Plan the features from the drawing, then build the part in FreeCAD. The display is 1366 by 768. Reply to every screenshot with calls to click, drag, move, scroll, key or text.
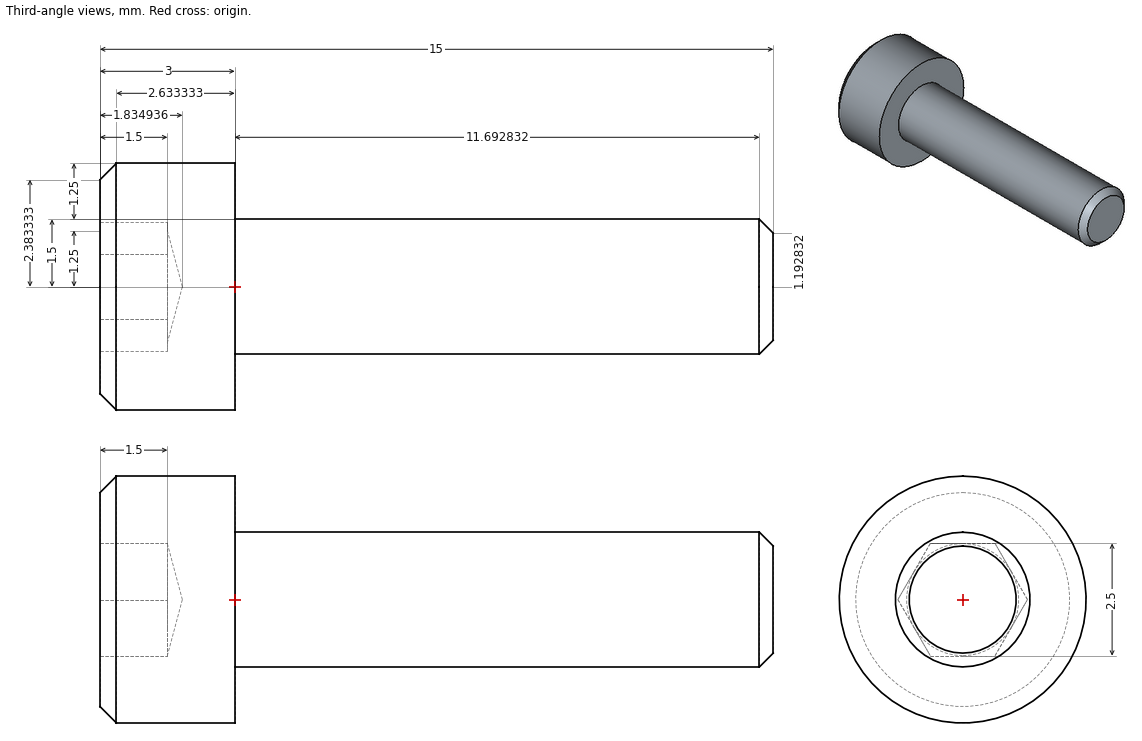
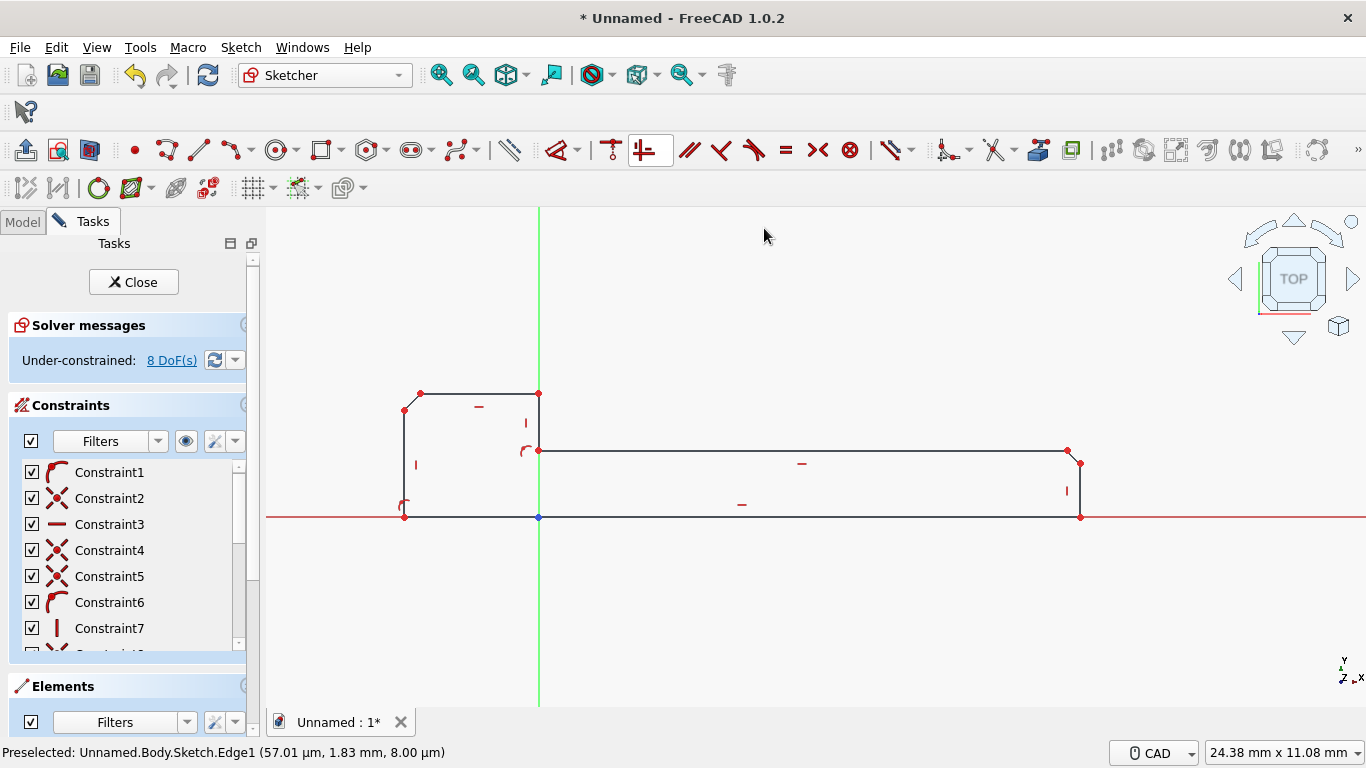
click(607, 517)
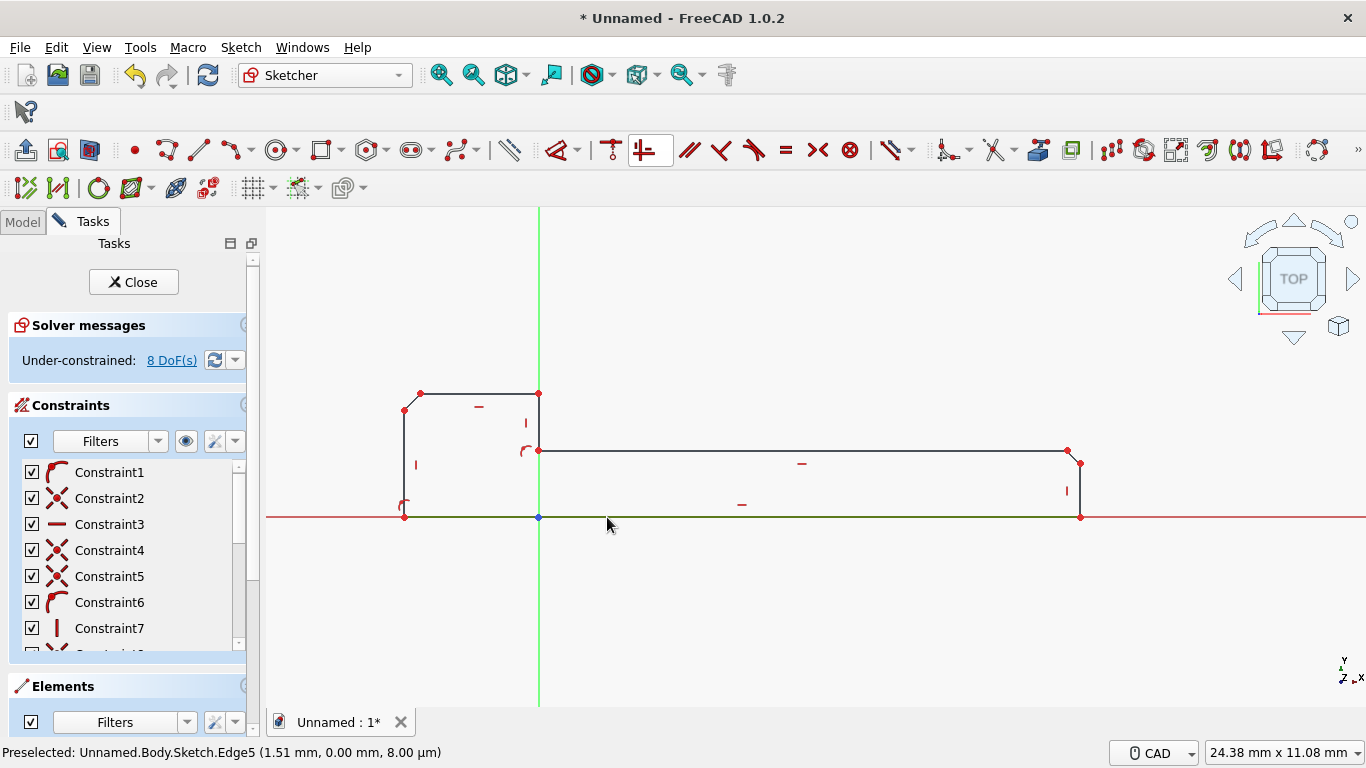
key(l)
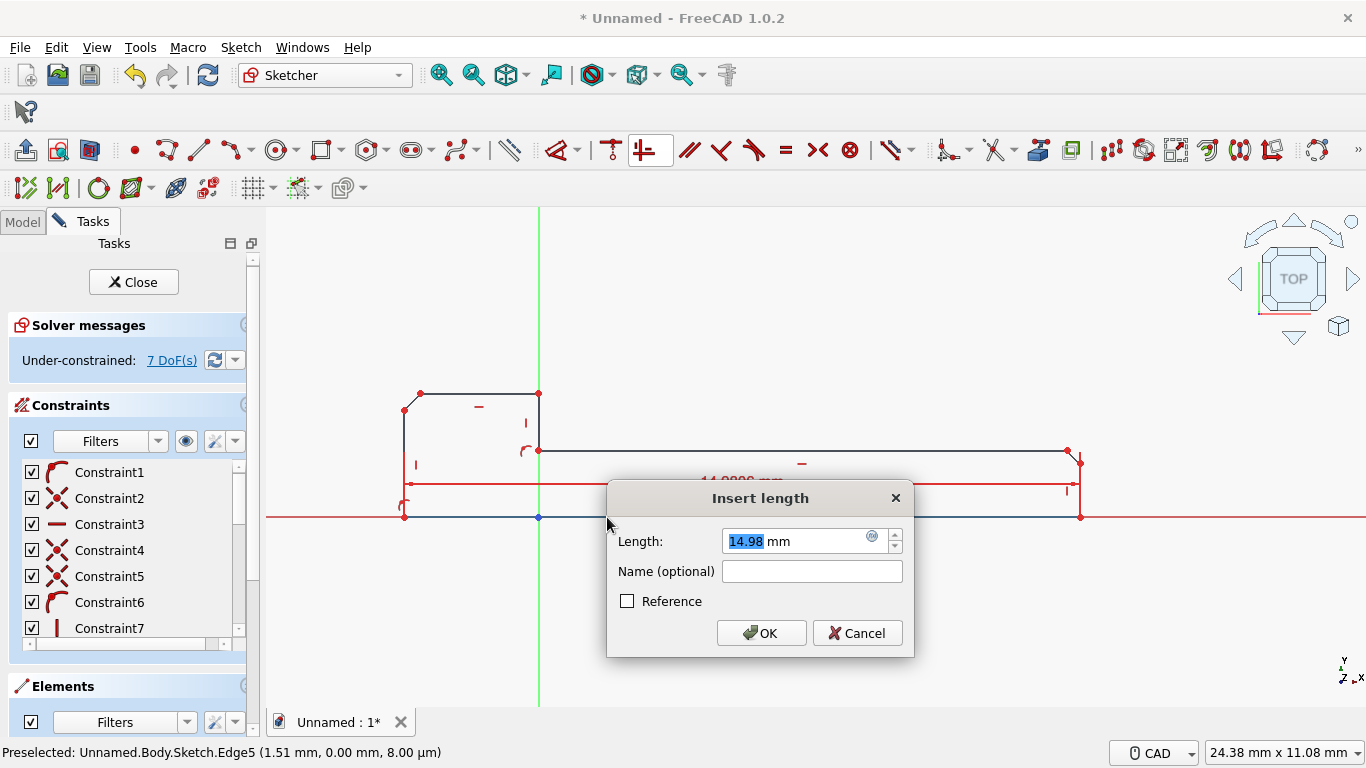
text(15)
key(Return)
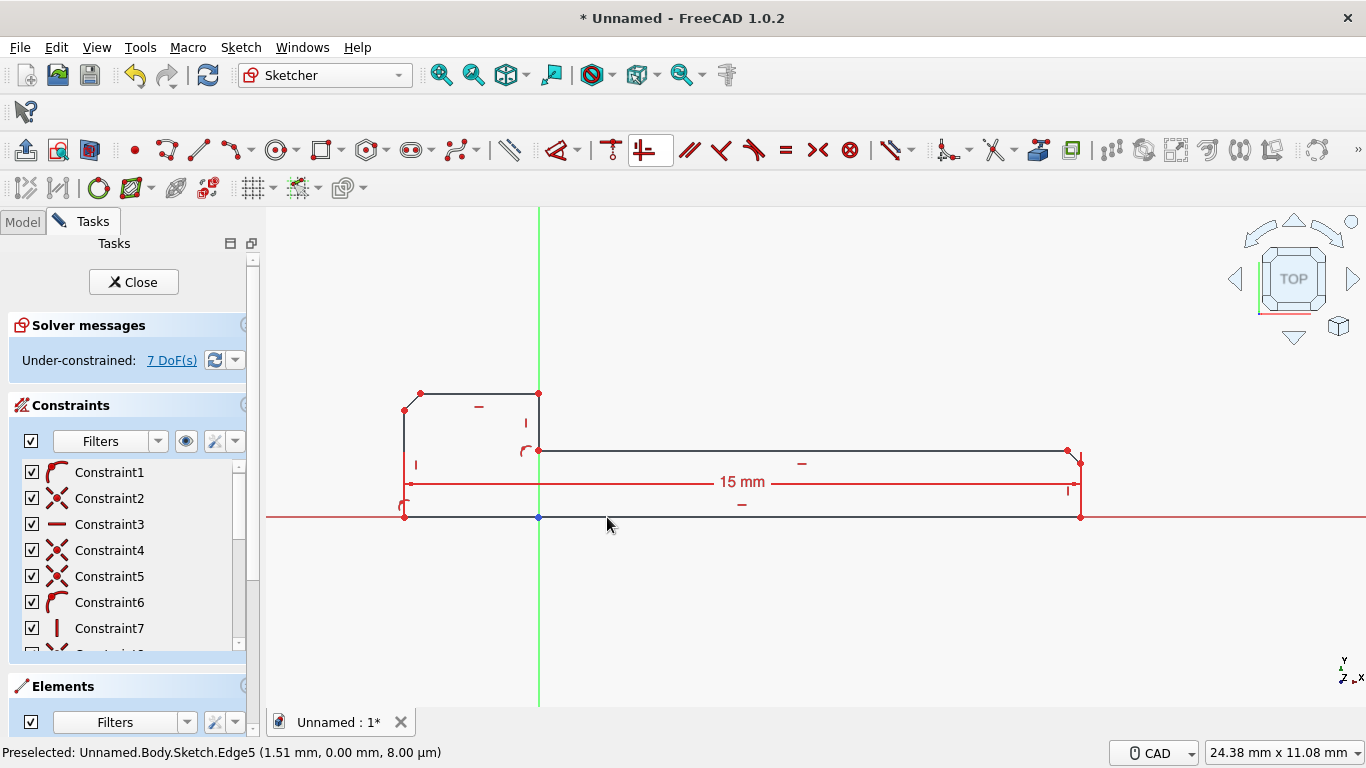
click(404, 411)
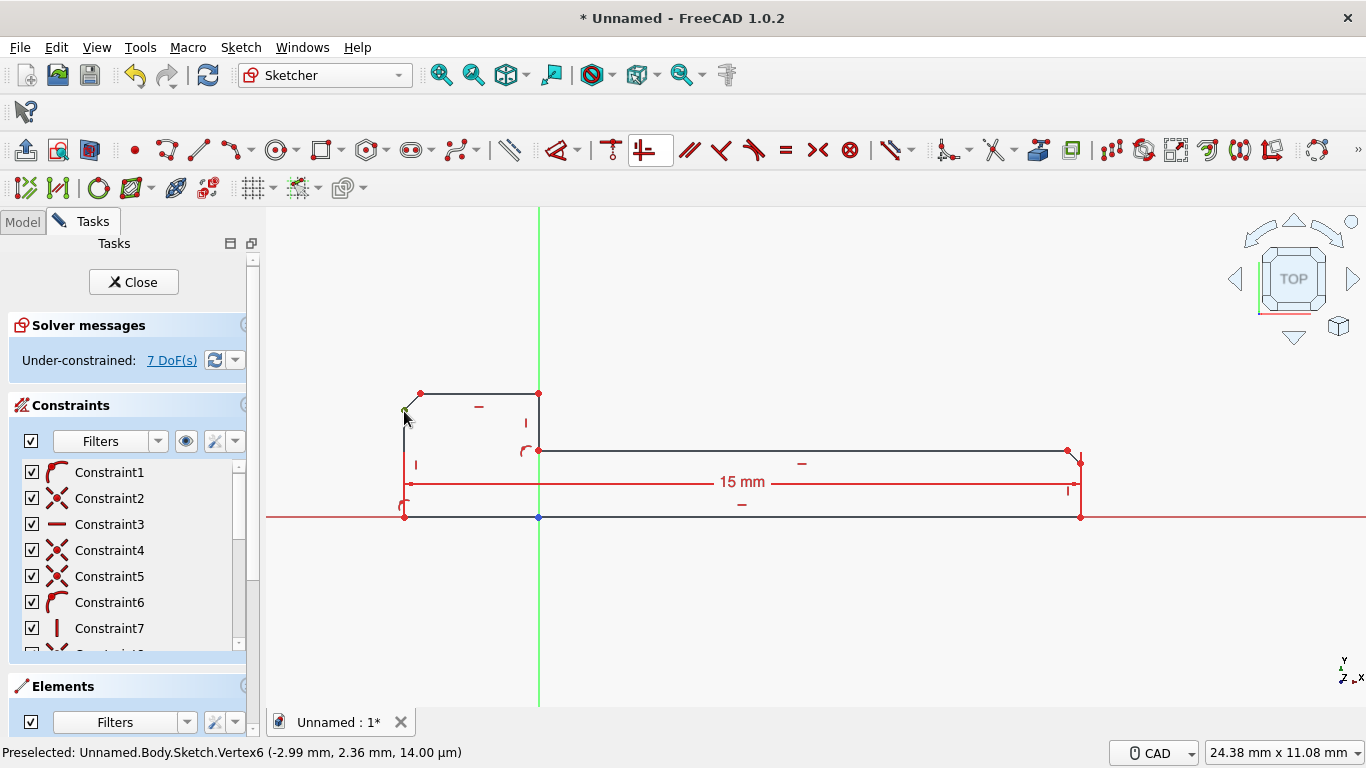
click(580, 150)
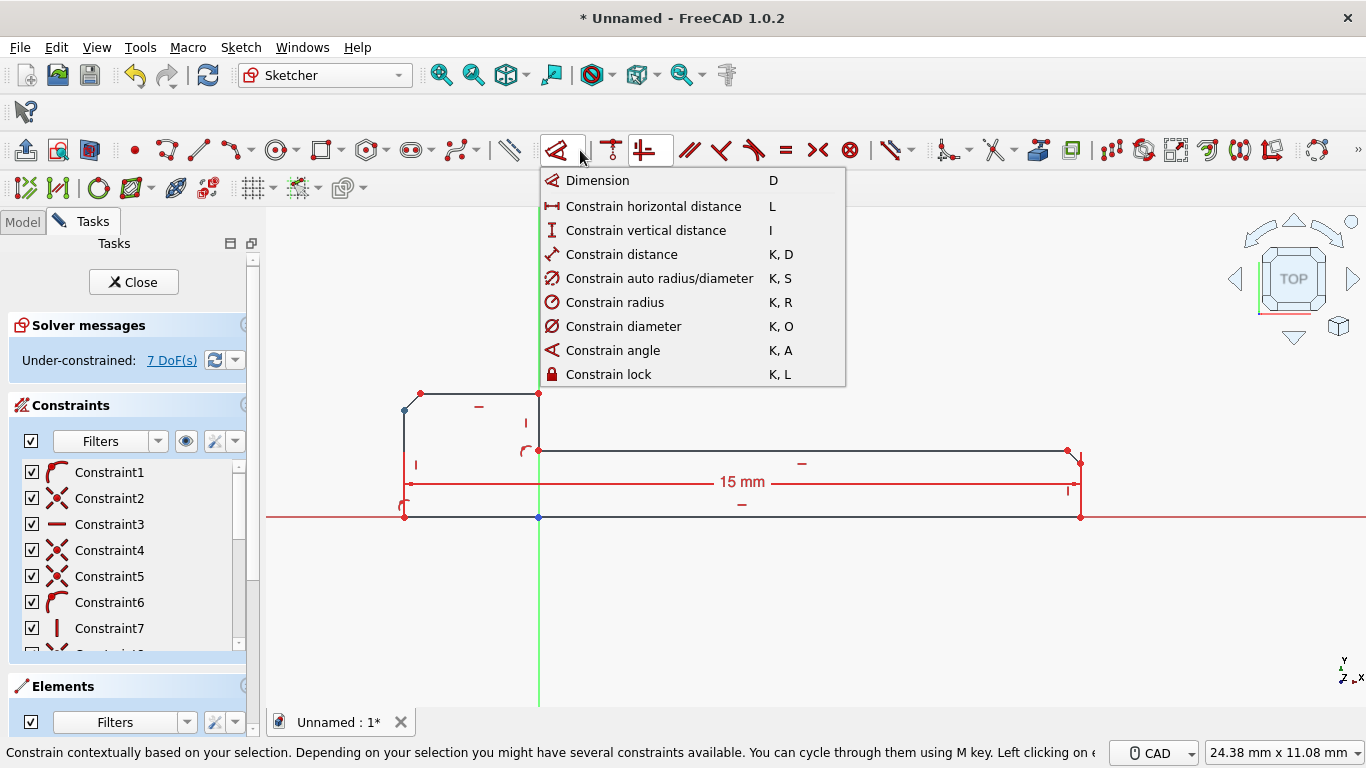
click(693, 206)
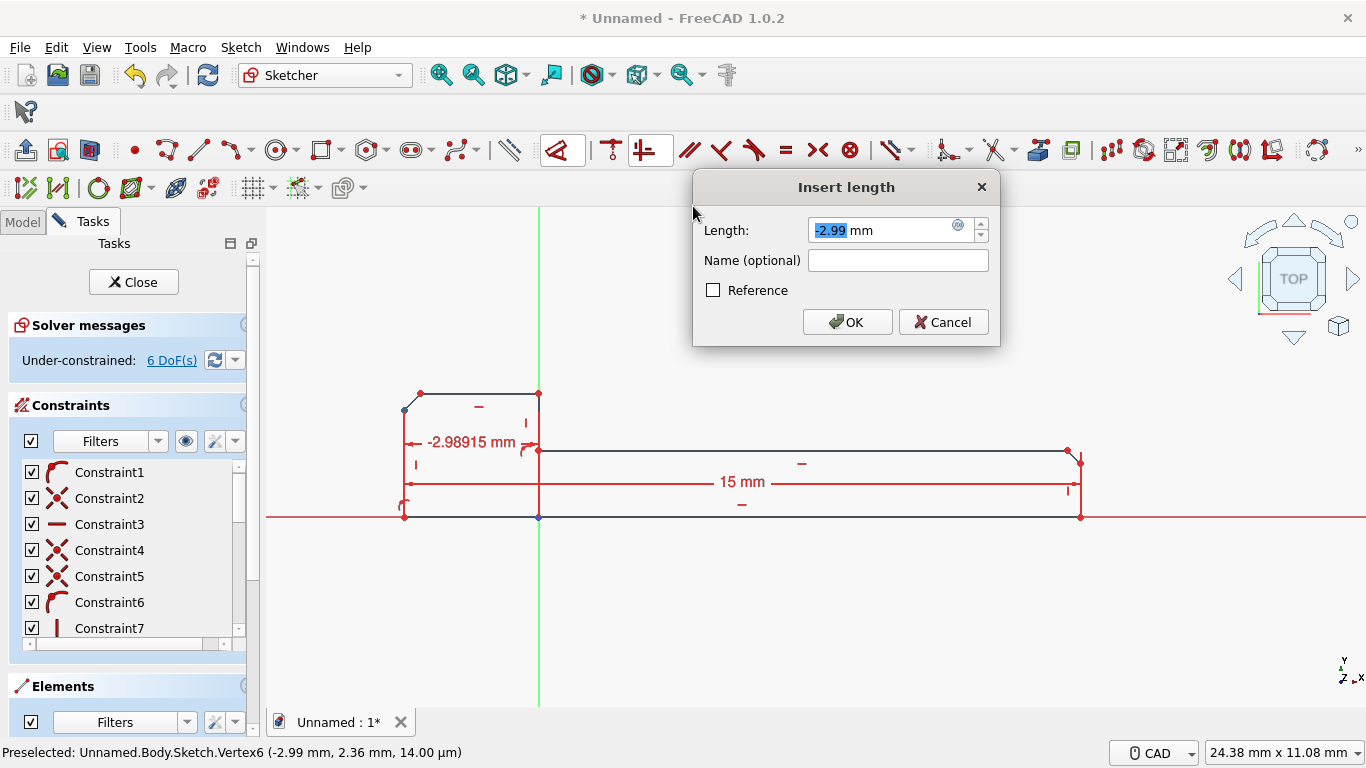
text(-3)
key(Return)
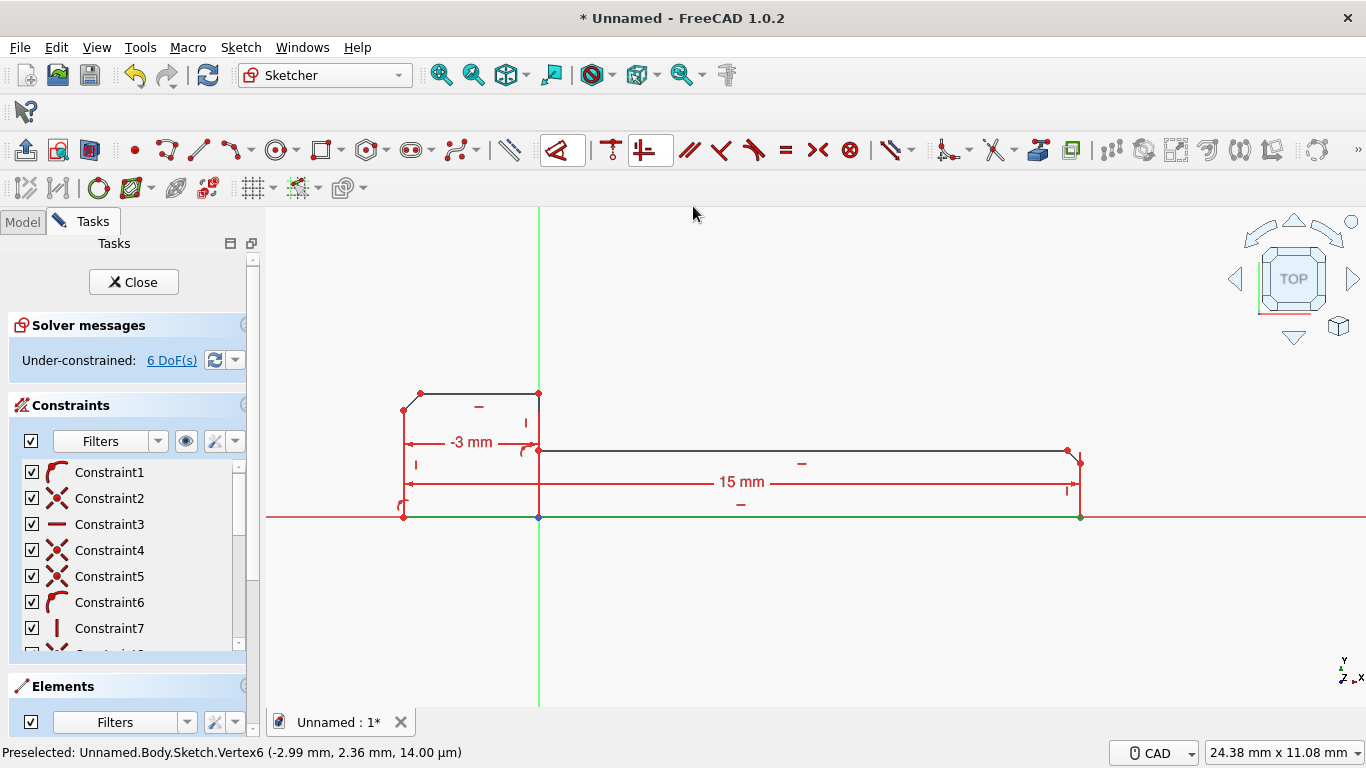
click(539, 434)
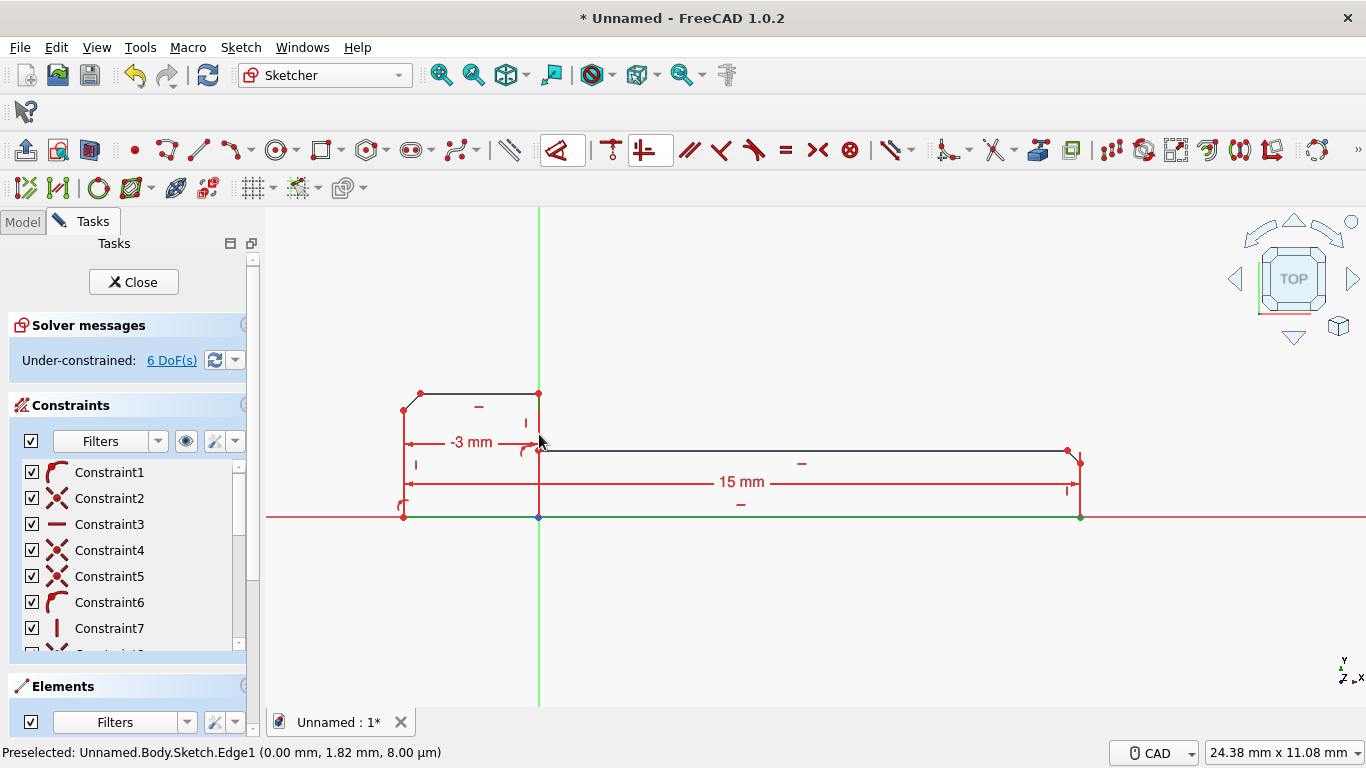
click(580, 150)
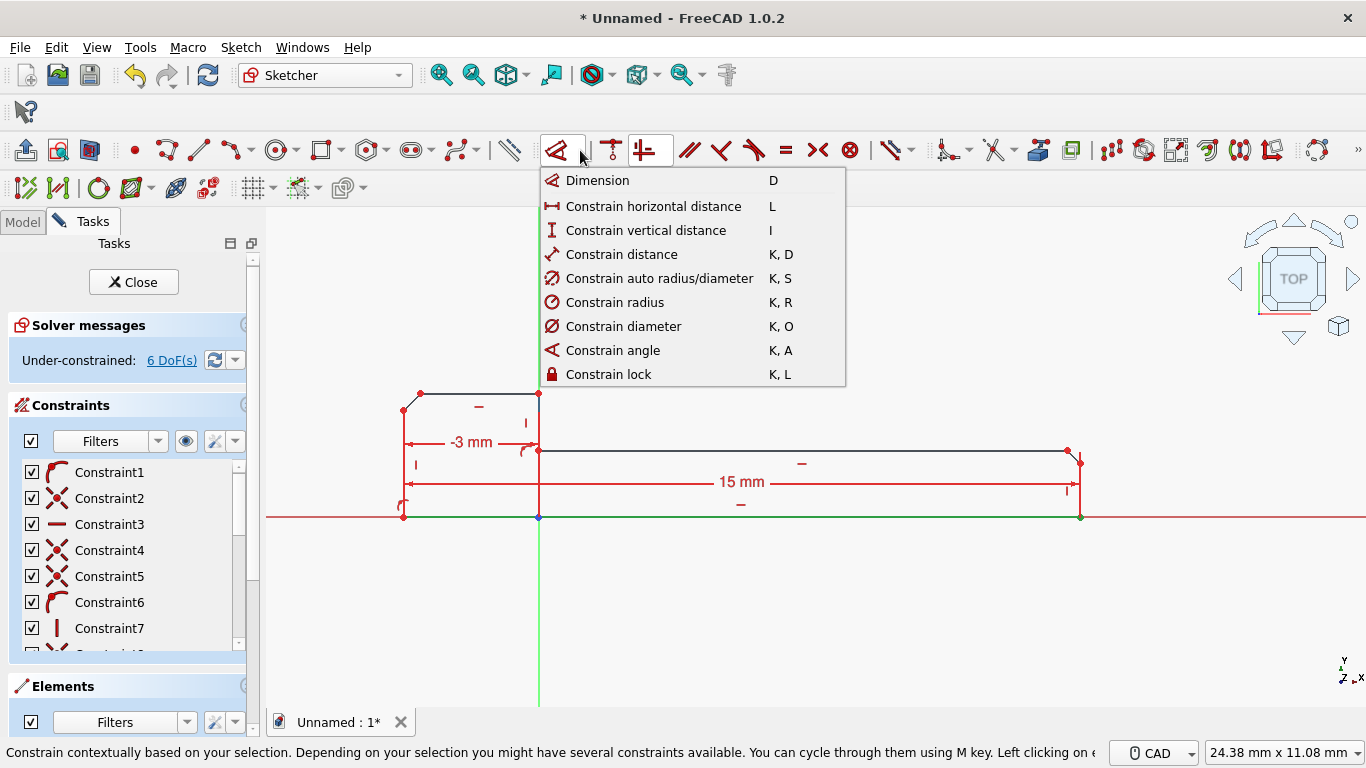
click(693, 230)